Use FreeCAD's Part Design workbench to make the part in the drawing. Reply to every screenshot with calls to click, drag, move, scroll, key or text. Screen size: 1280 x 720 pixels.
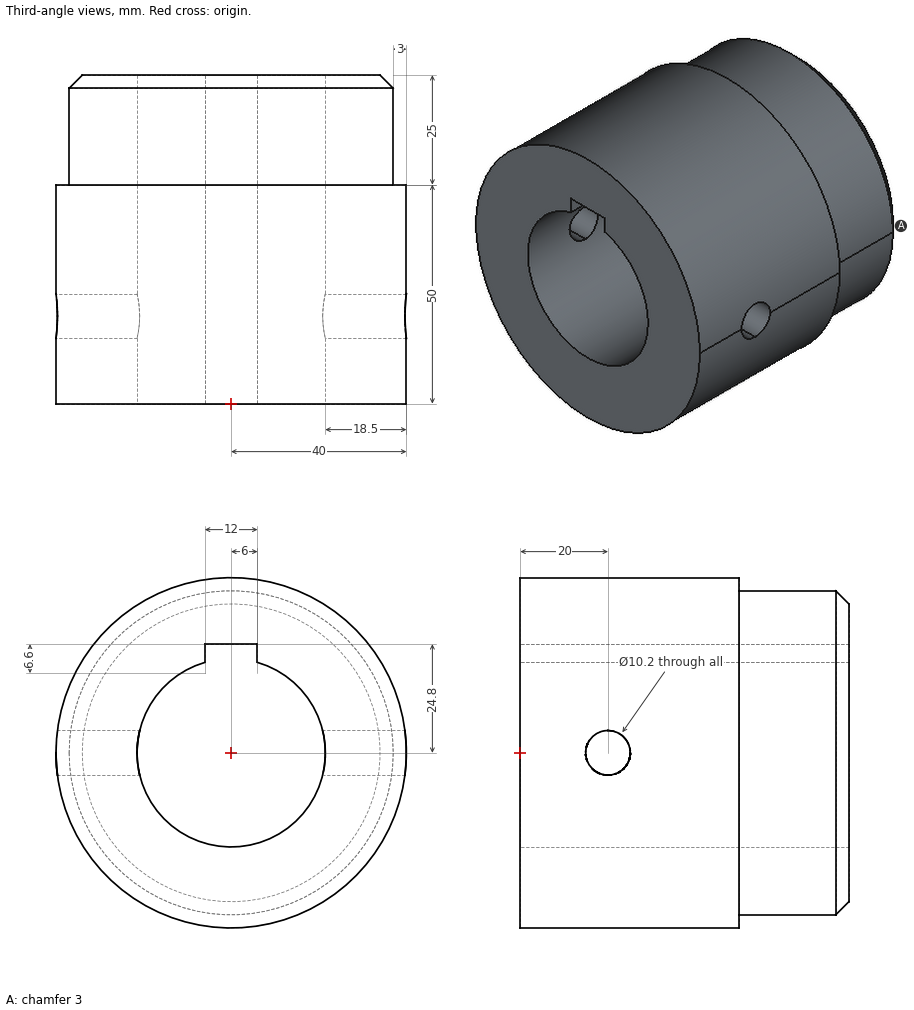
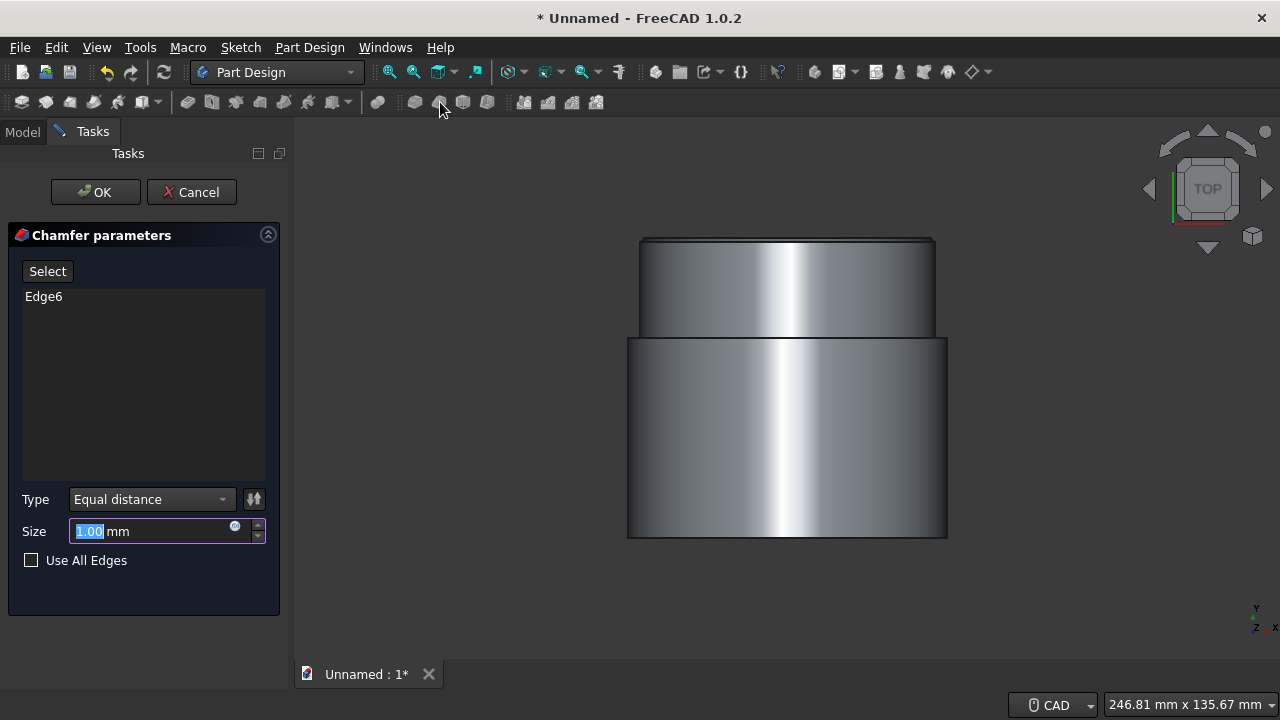
text(3)
key(Tab)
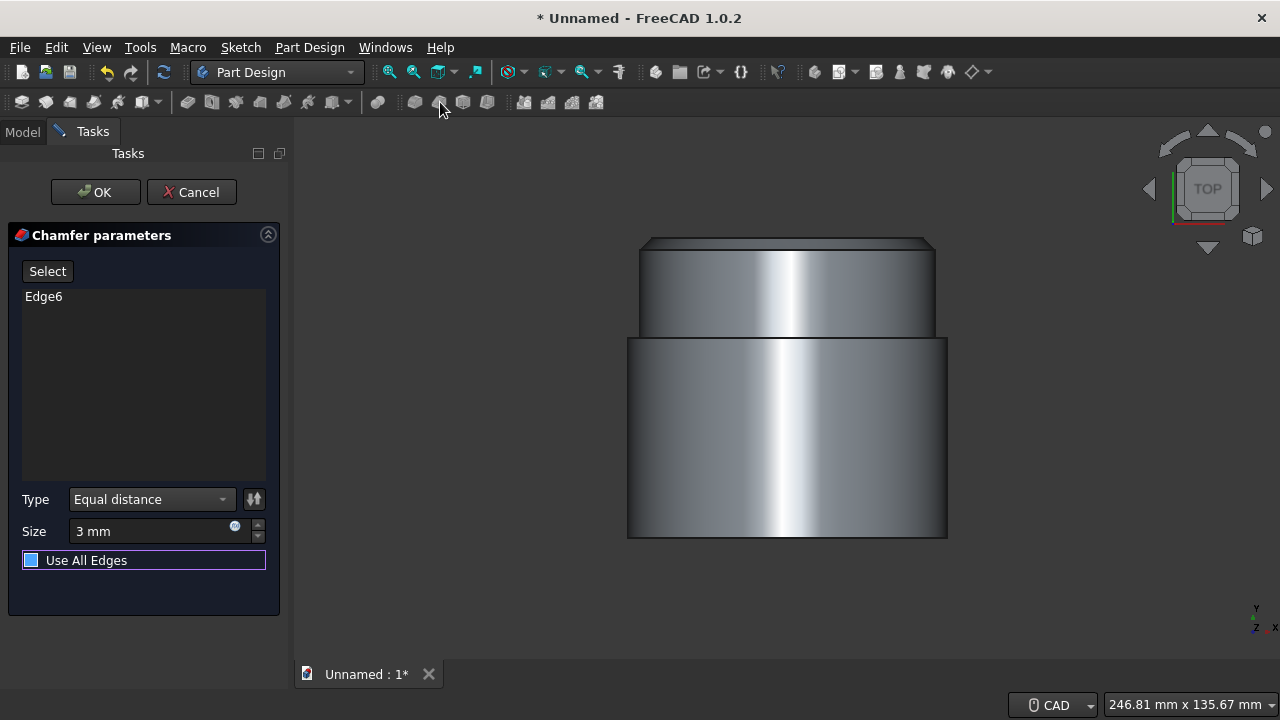
click(96, 192)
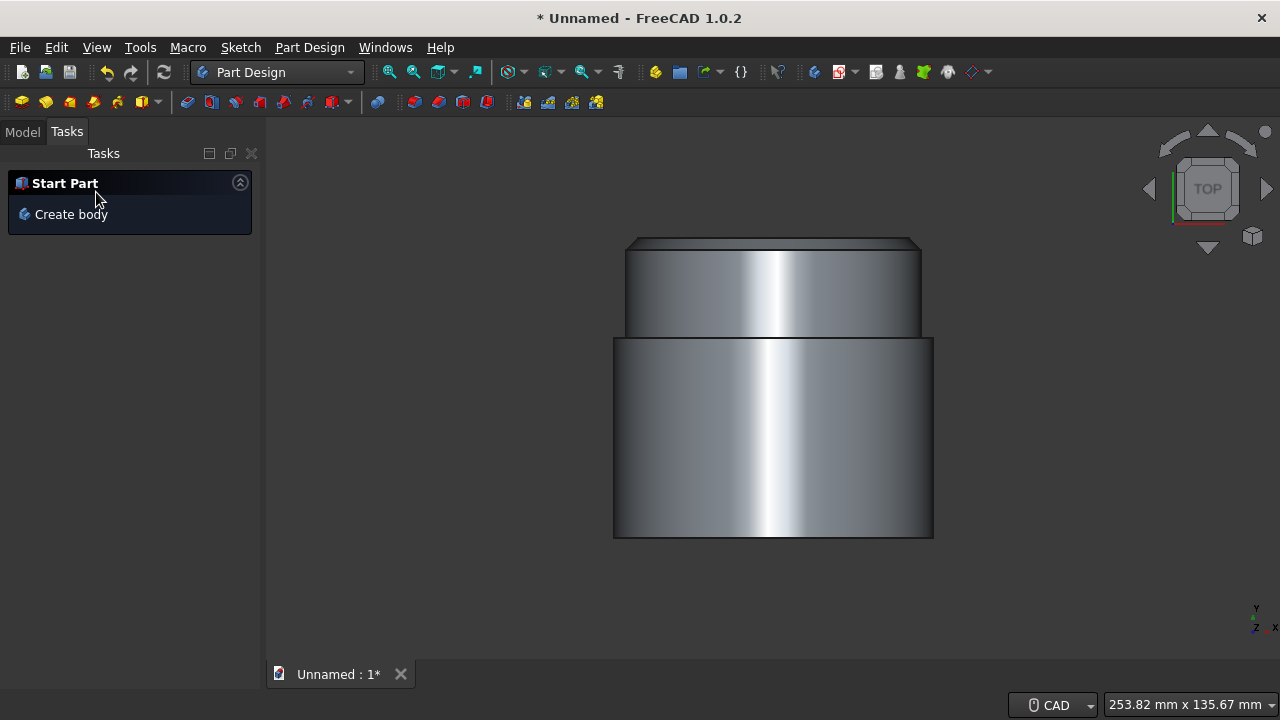
click(23, 131)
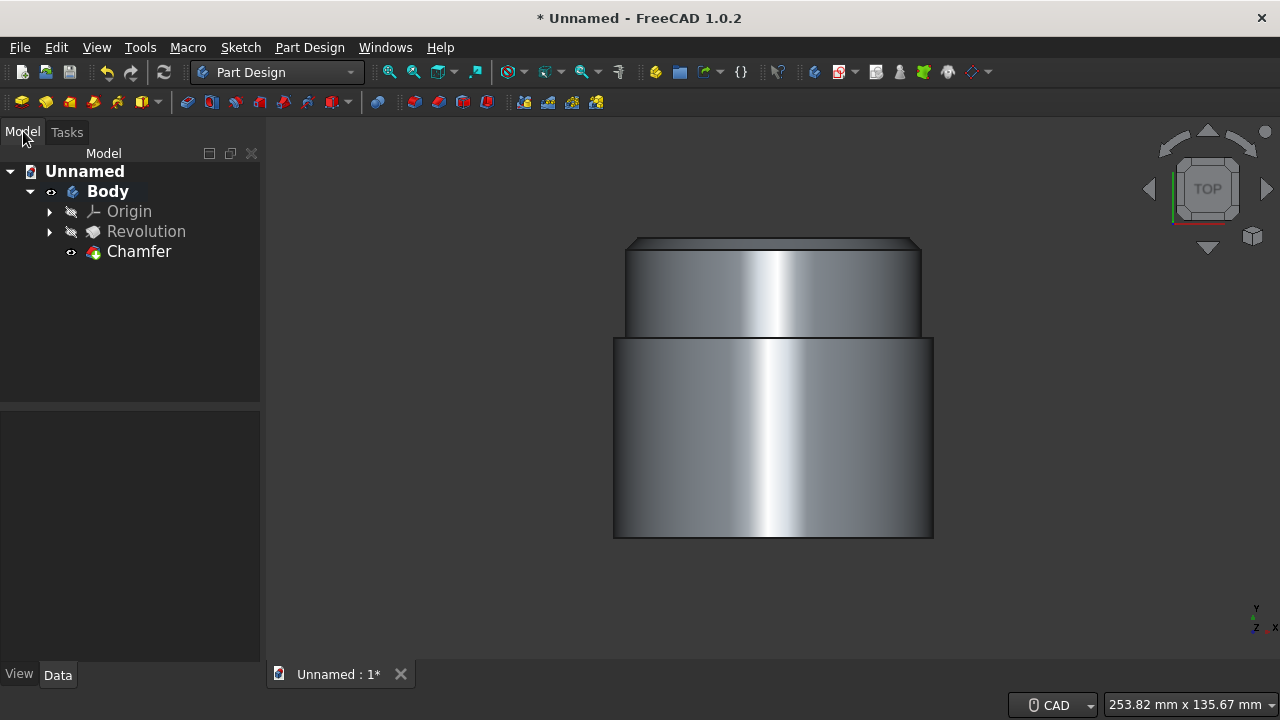
click(50, 212)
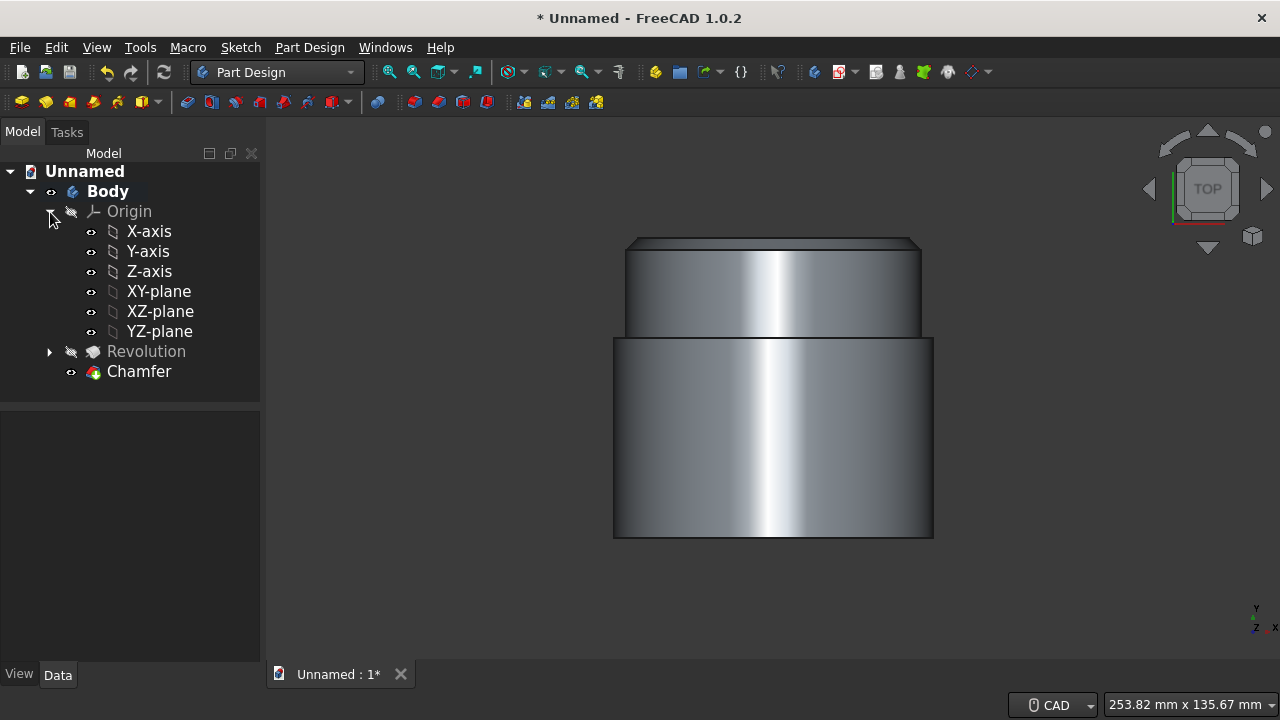
click(136, 332)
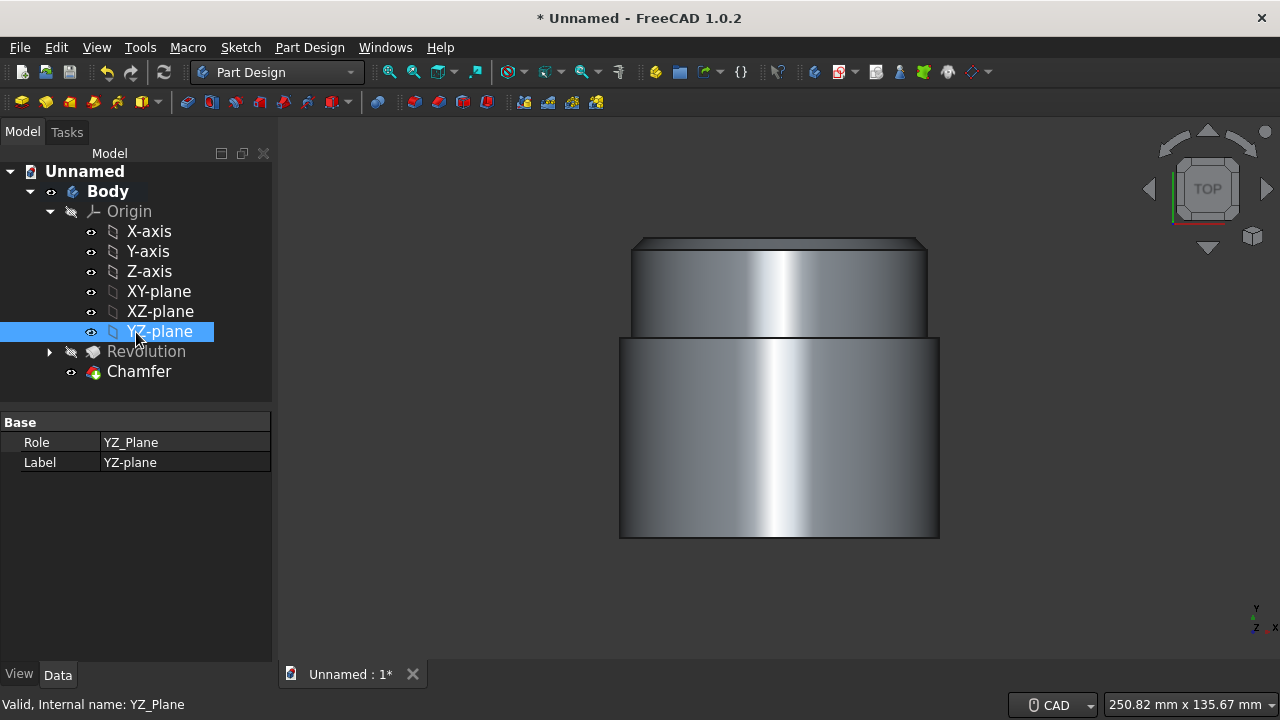
click(972, 72)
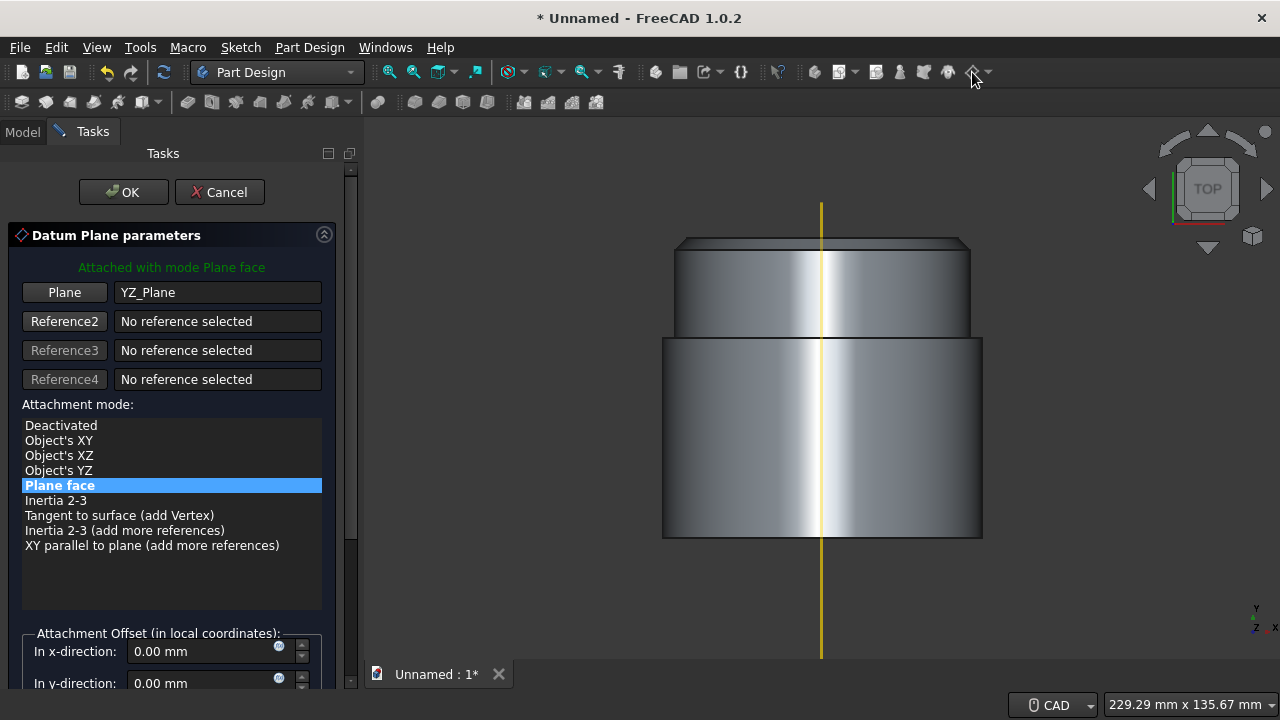
scroll(351, 426, down, 2)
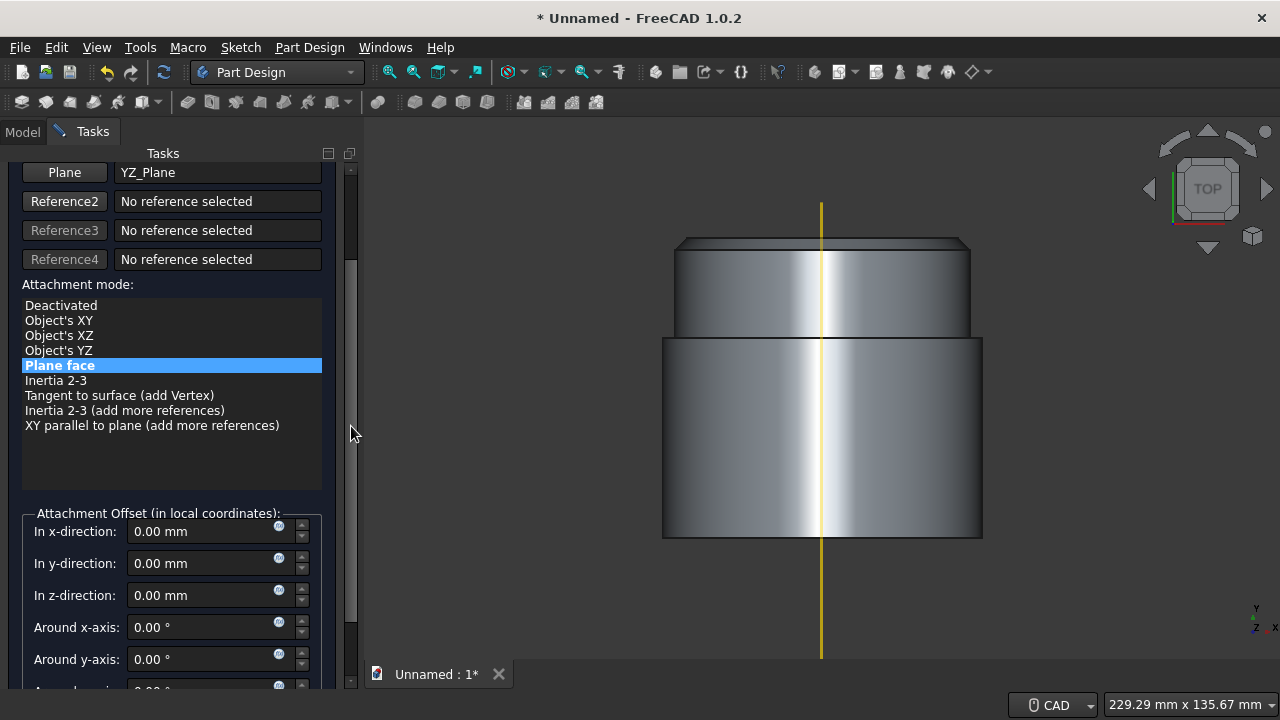
triple_click(210, 595)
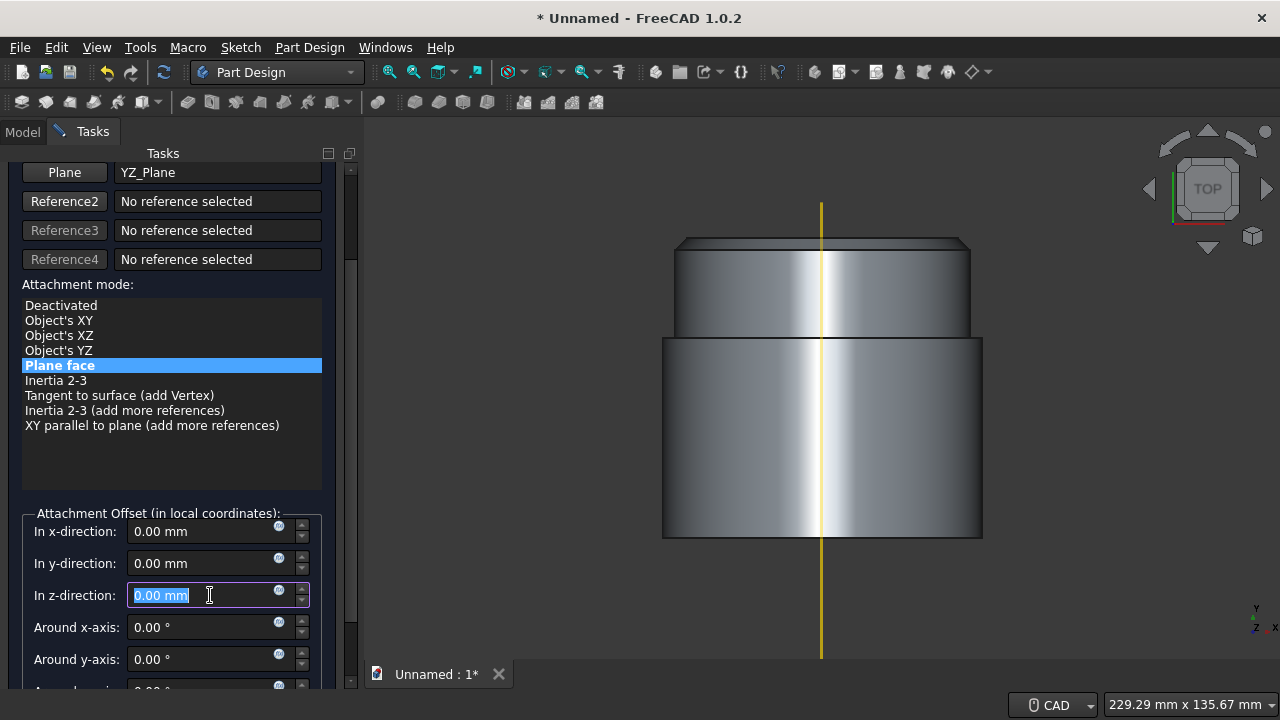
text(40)
key(Tab)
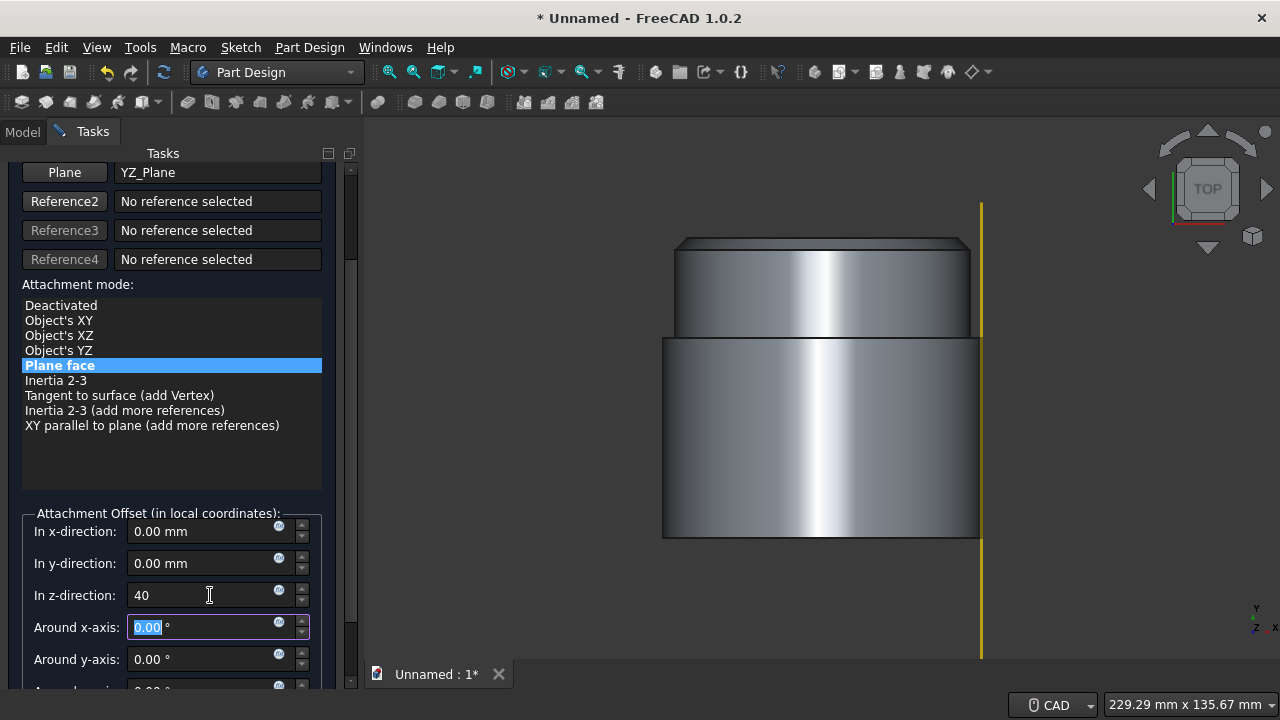
scroll(351, 426, up, 3)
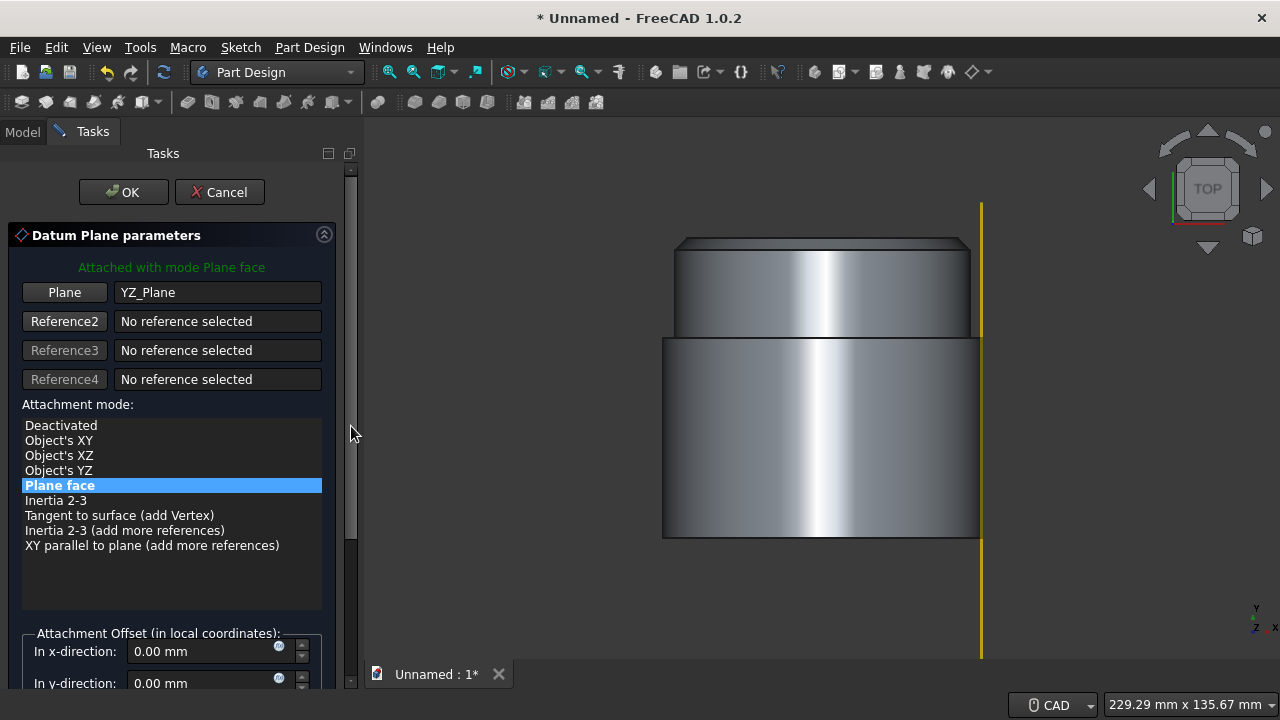
click(124, 192)